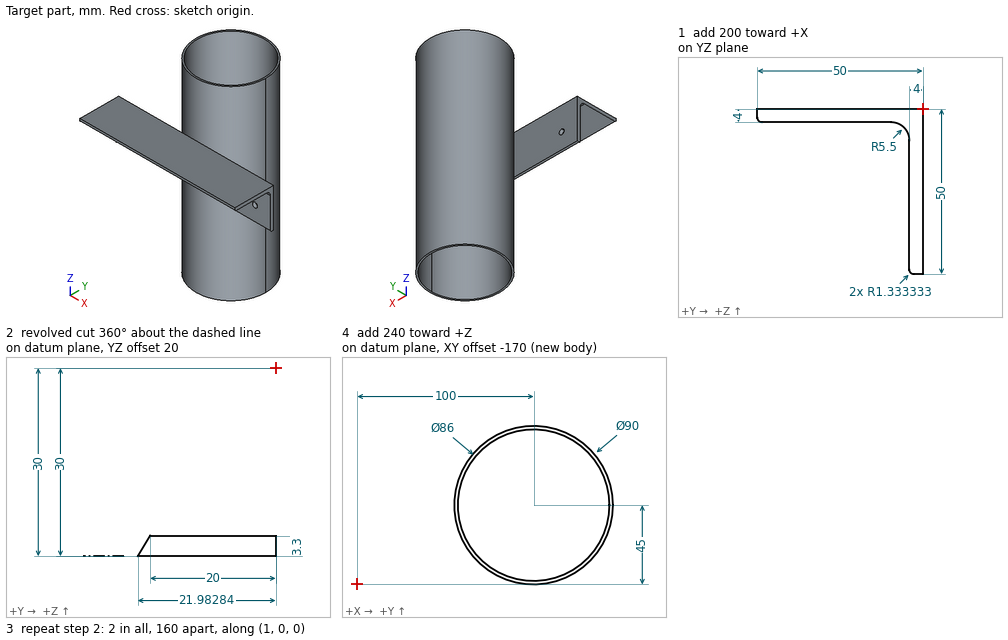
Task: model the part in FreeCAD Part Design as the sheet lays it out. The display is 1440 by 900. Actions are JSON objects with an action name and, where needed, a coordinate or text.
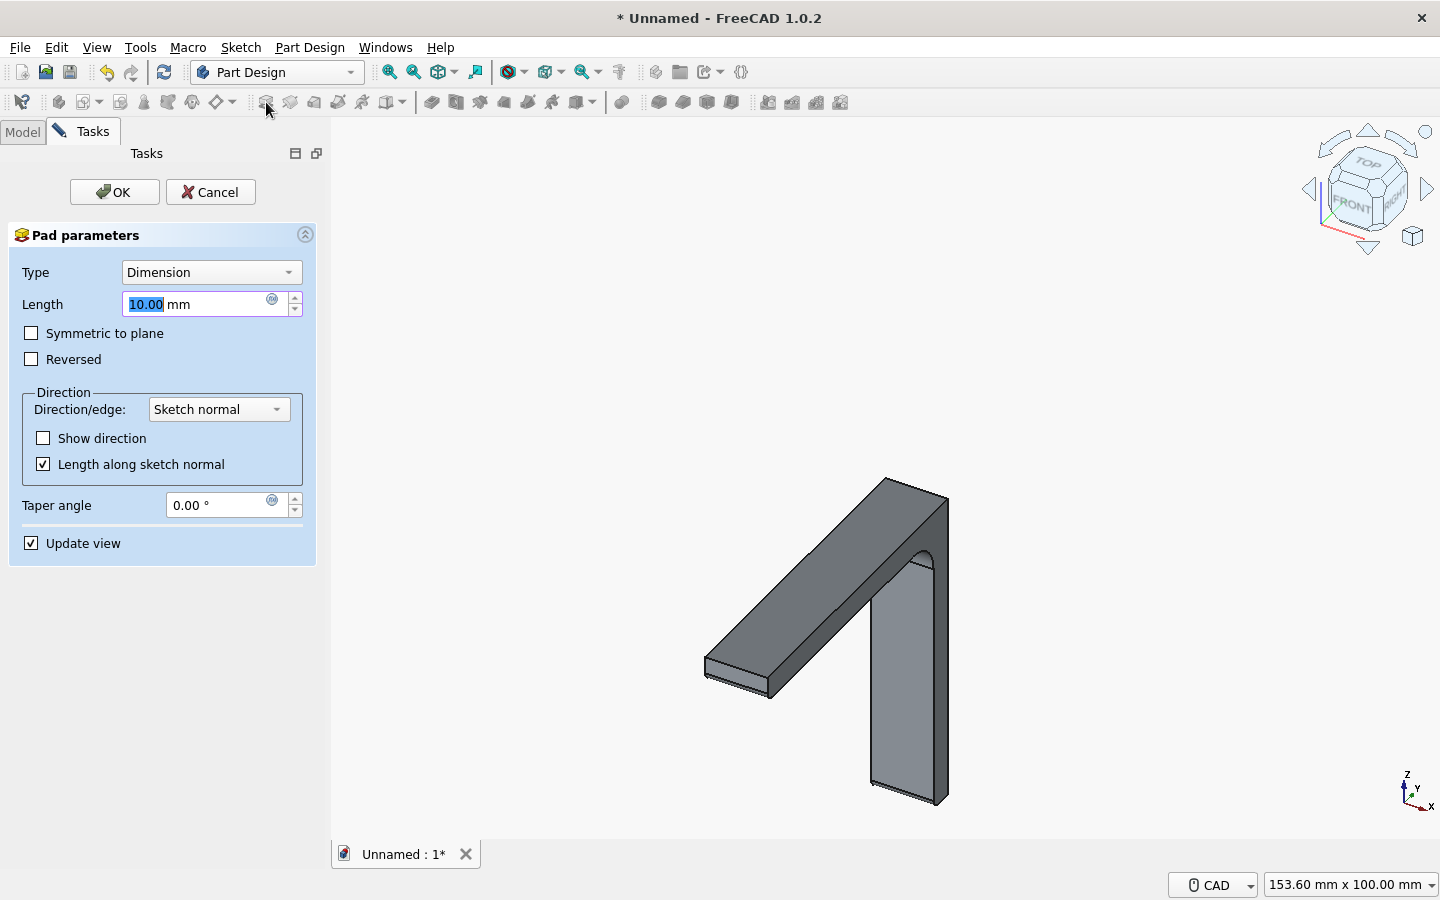
{"action": "type", "text": "200"}
{"action": "key", "text": "Tab"}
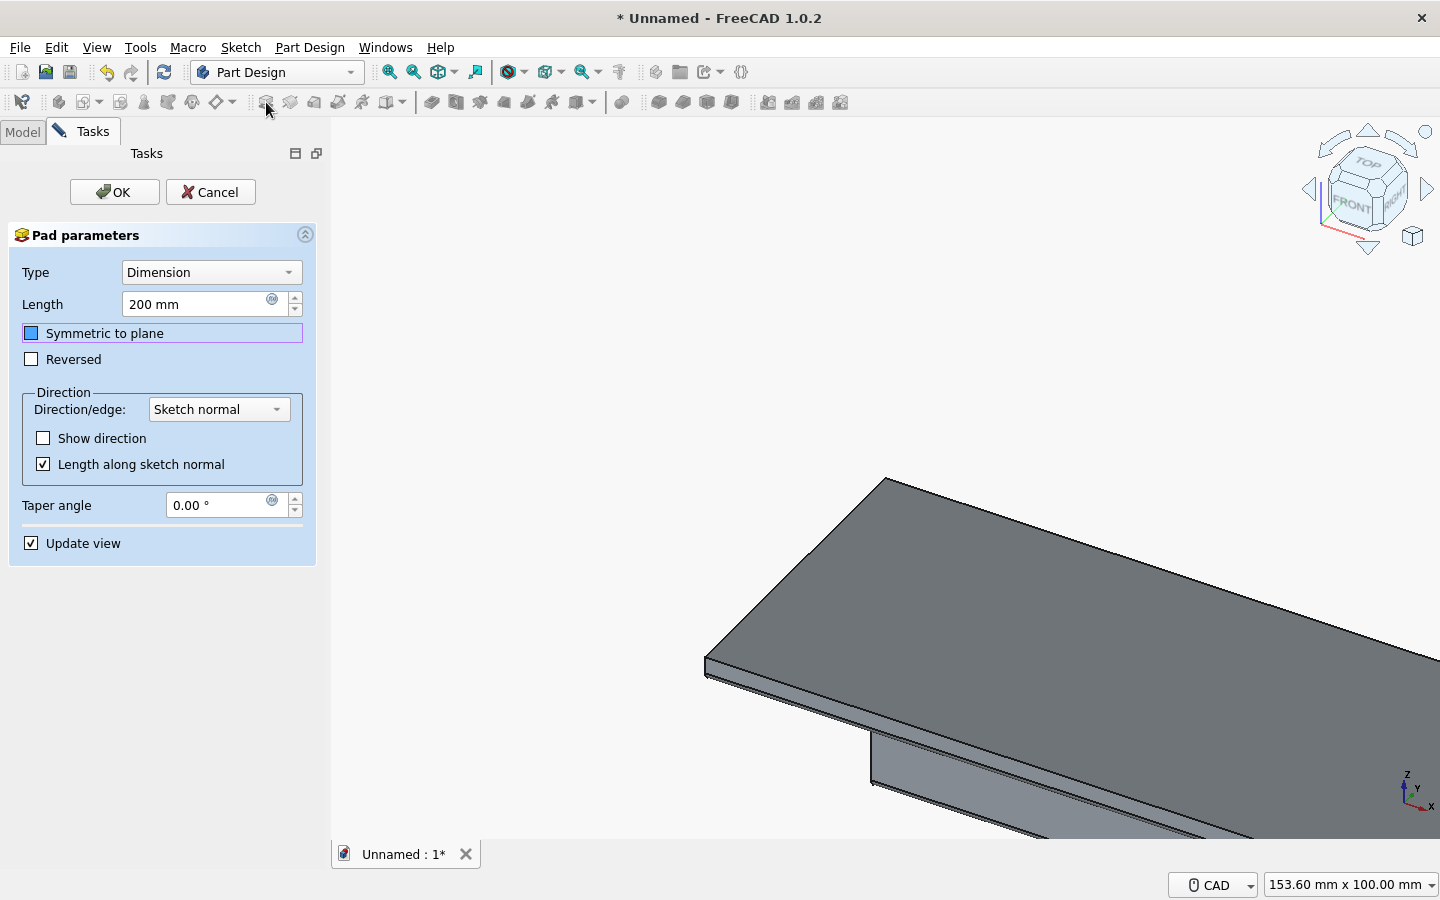
{"action": "left_click", "coordinate": [115, 192]}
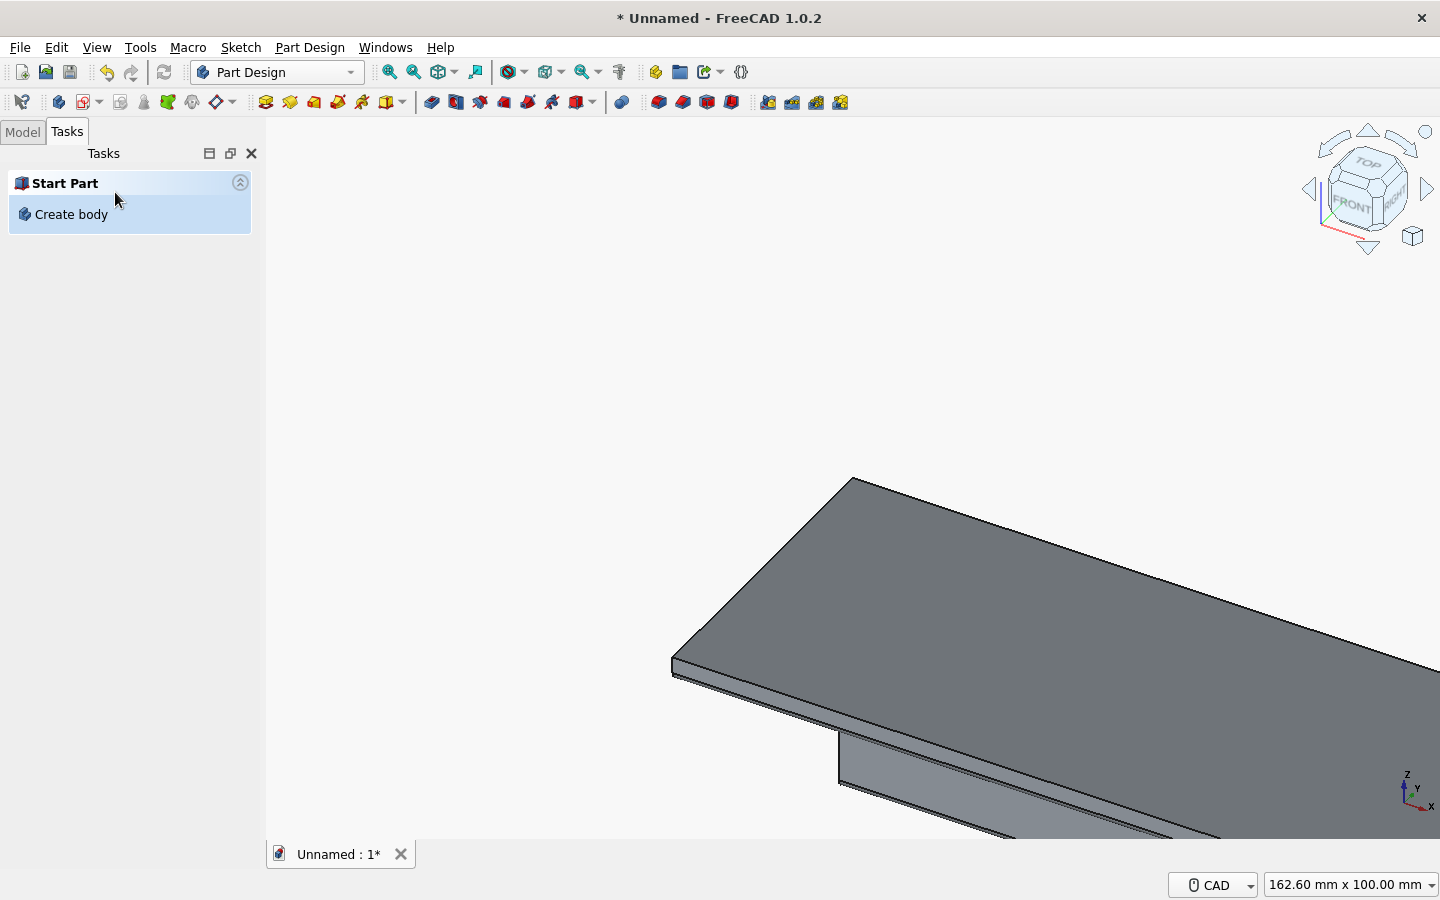
{"action": "left_click", "coordinate": [390, 72]}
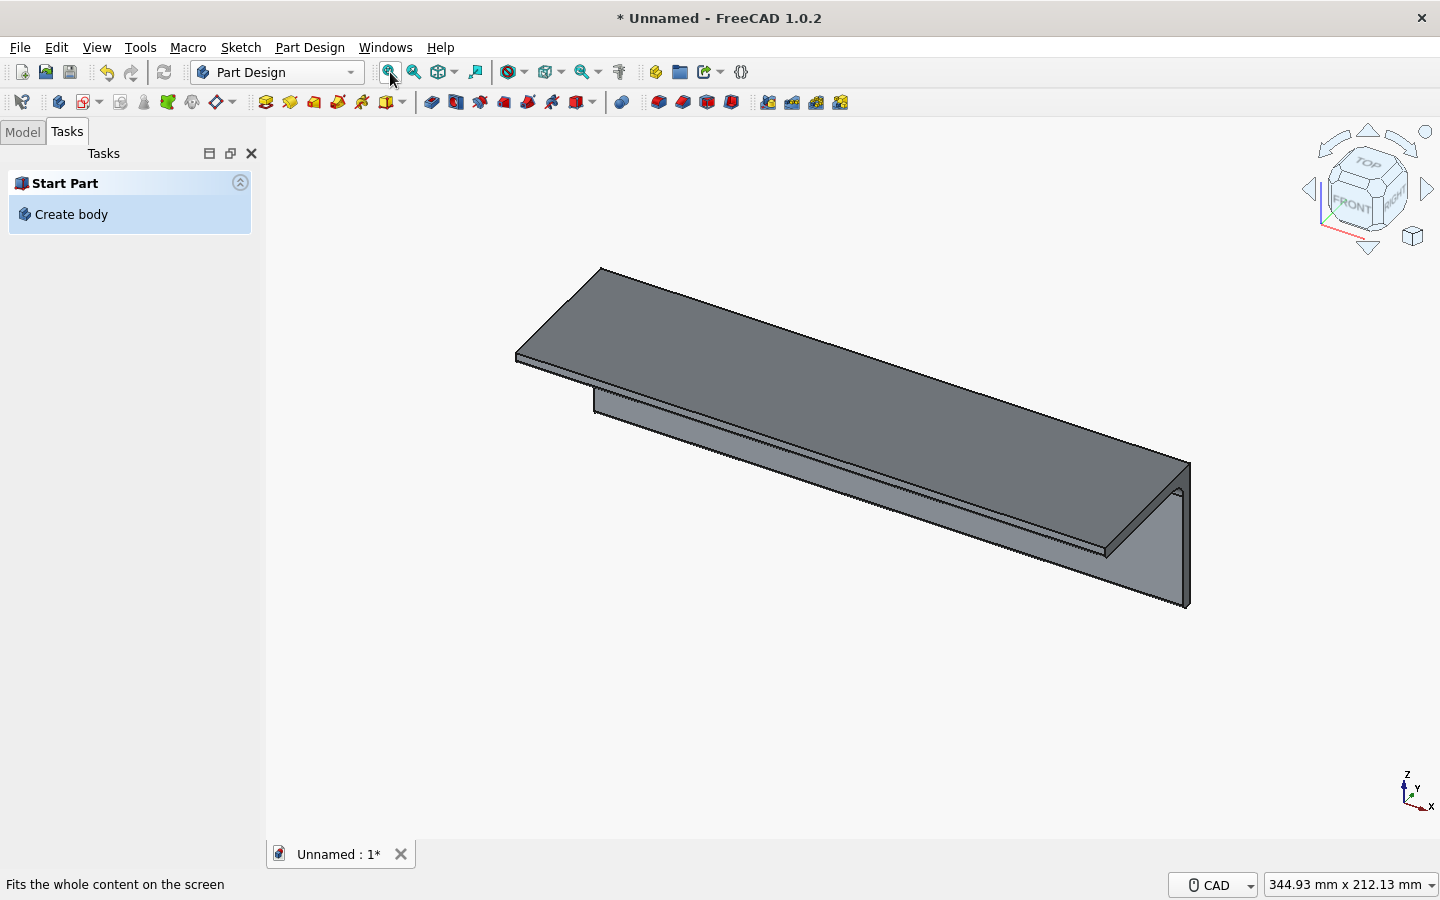
{"action": "left_click", "coordinate": [23, 131]}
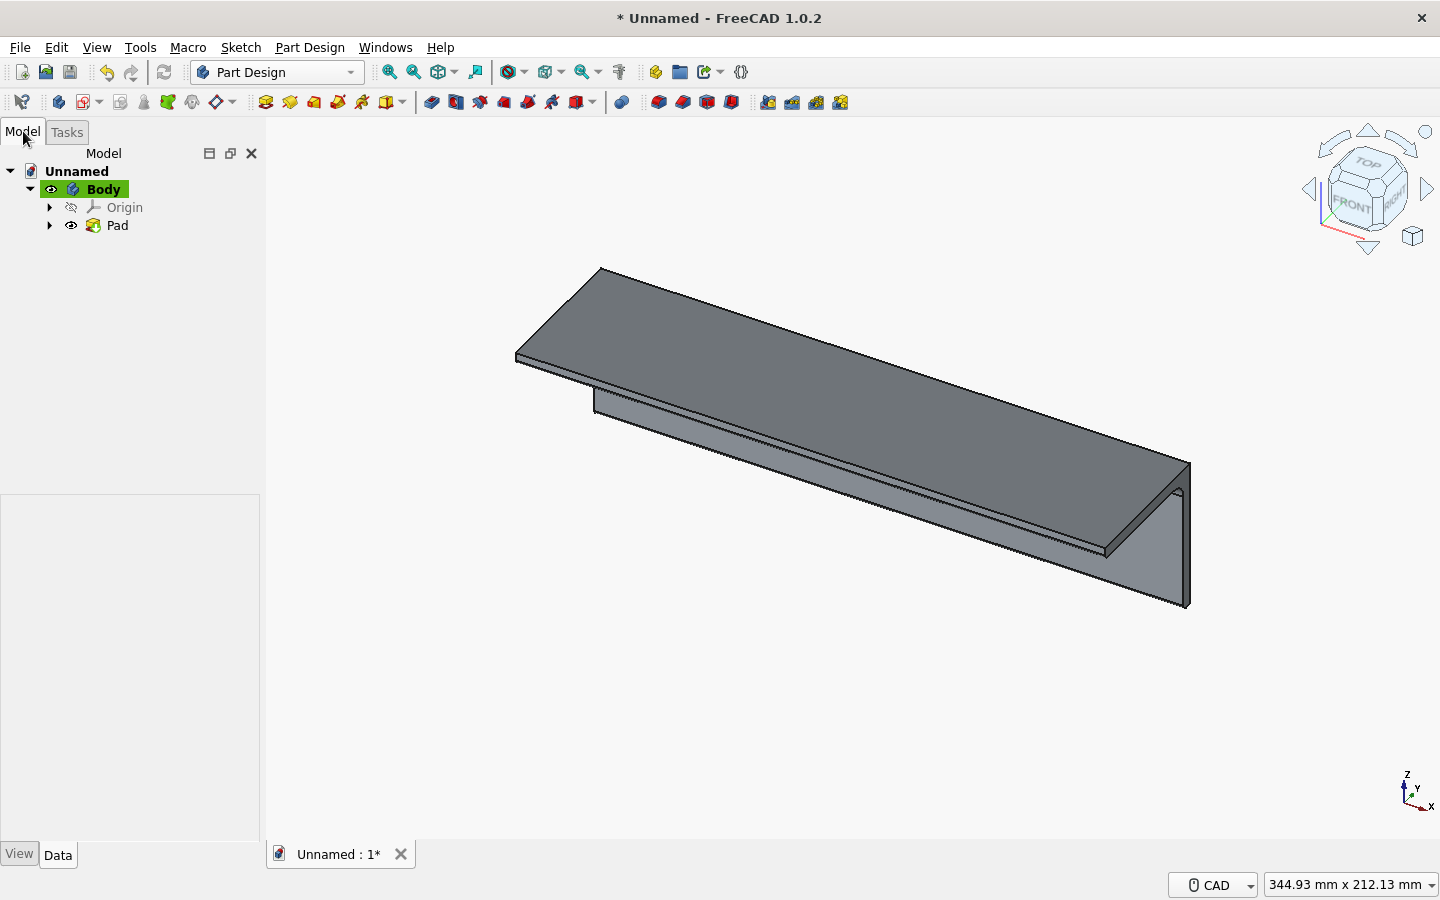
{"action": "left_click", "coordinate": [50, 207]}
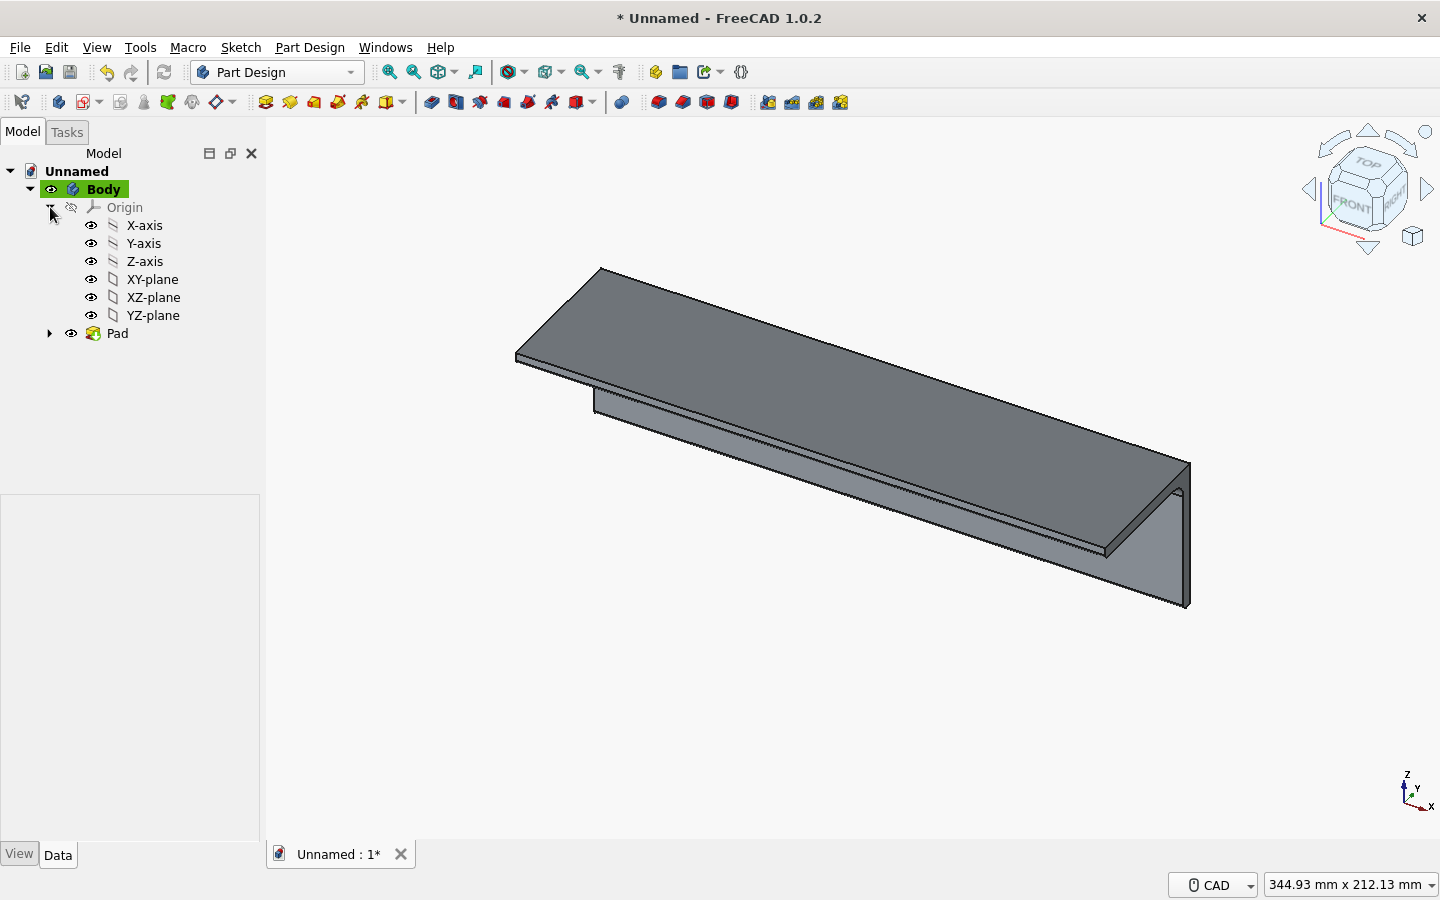
{"action": "left_click", "coordinate": [136, 315]}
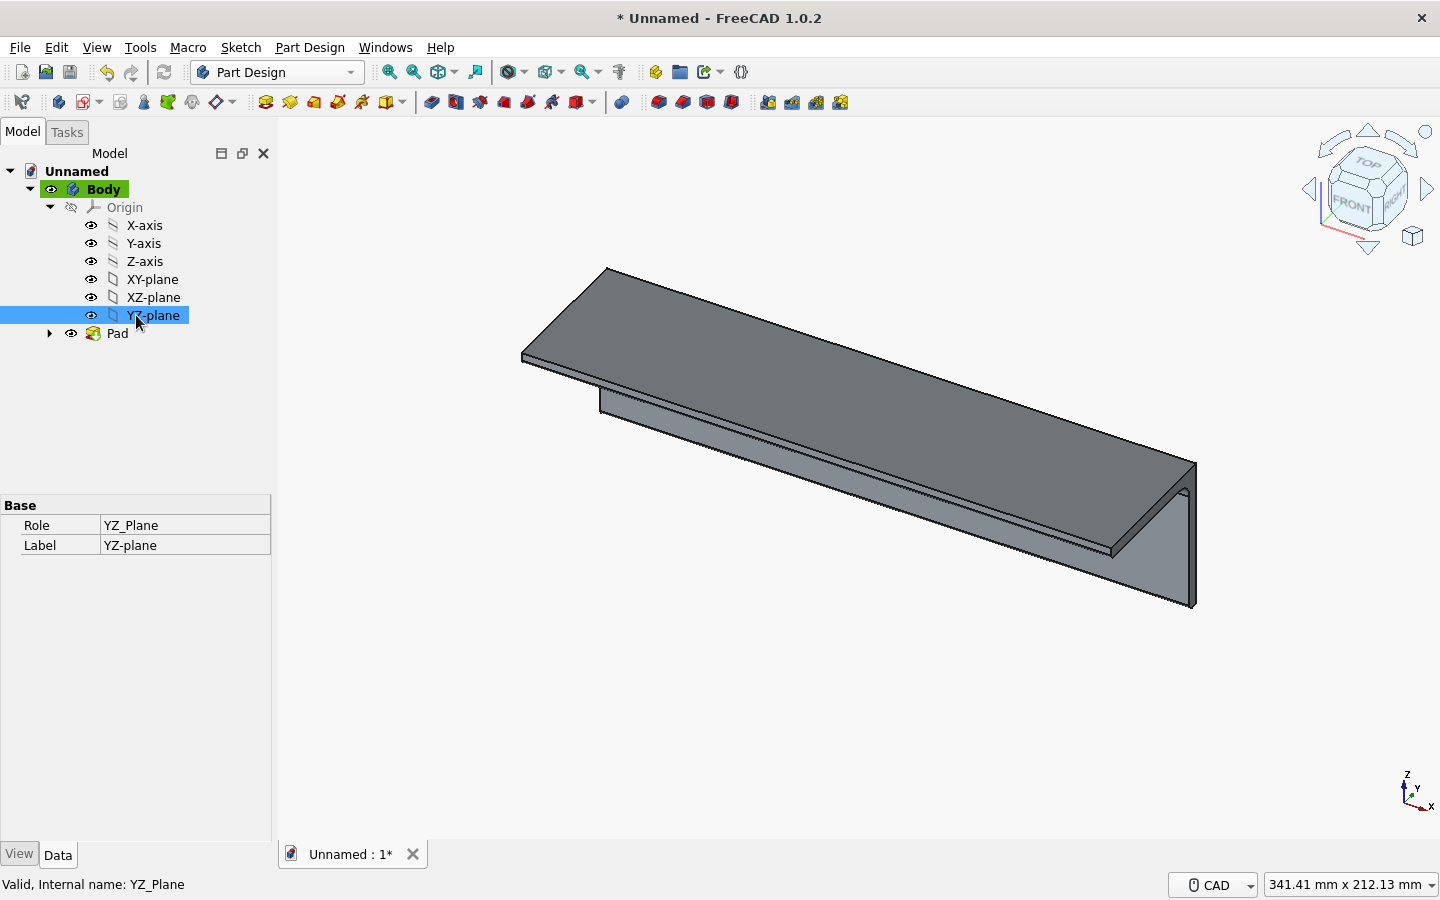
{"action": "left_click", "coordinate": [216, 102]}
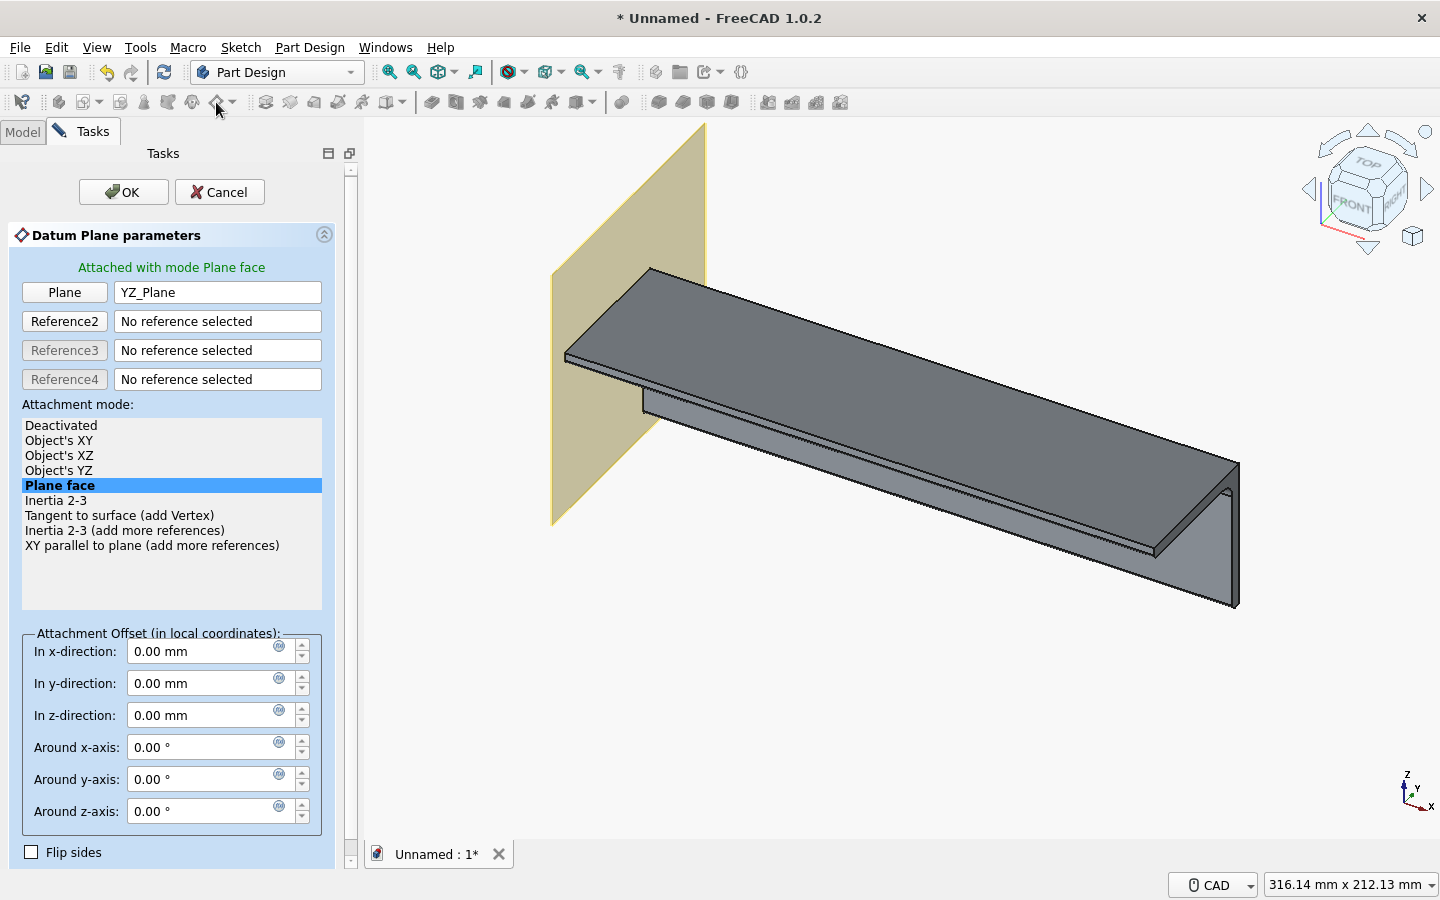
{"action": "triple_click", "coordinate": [210, 715]}